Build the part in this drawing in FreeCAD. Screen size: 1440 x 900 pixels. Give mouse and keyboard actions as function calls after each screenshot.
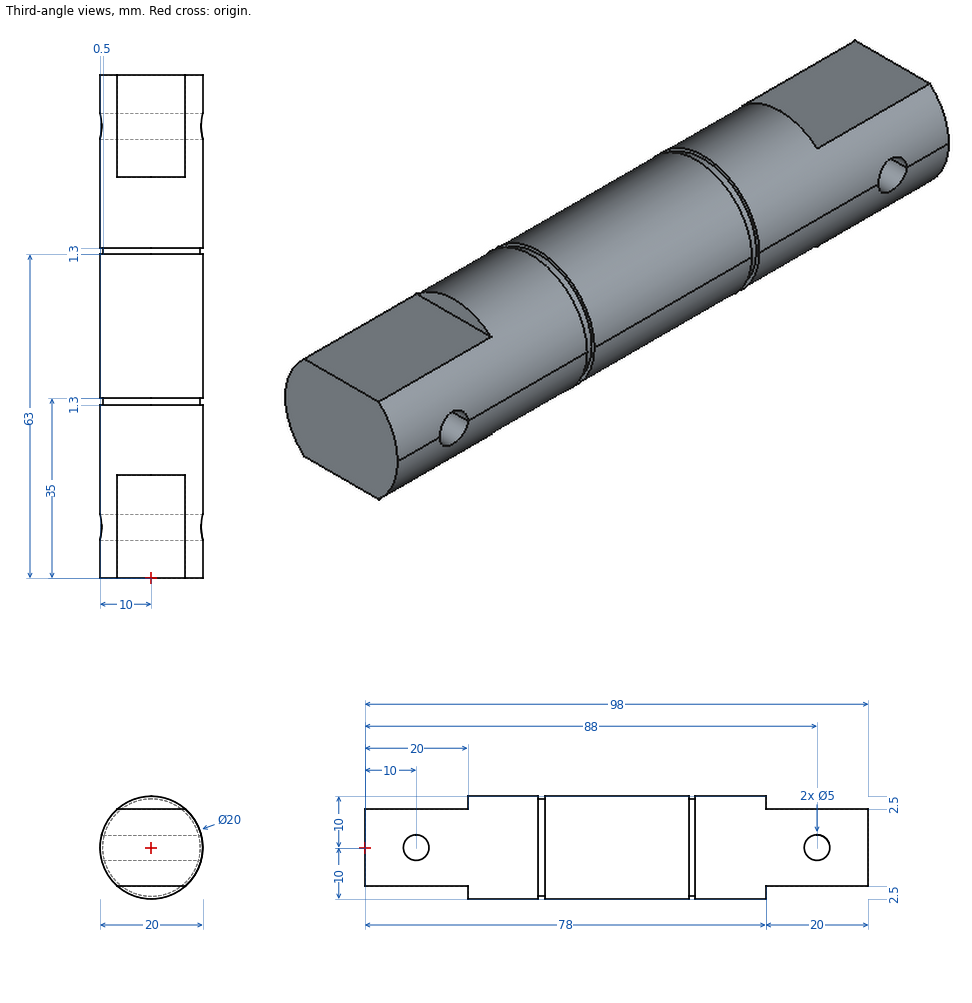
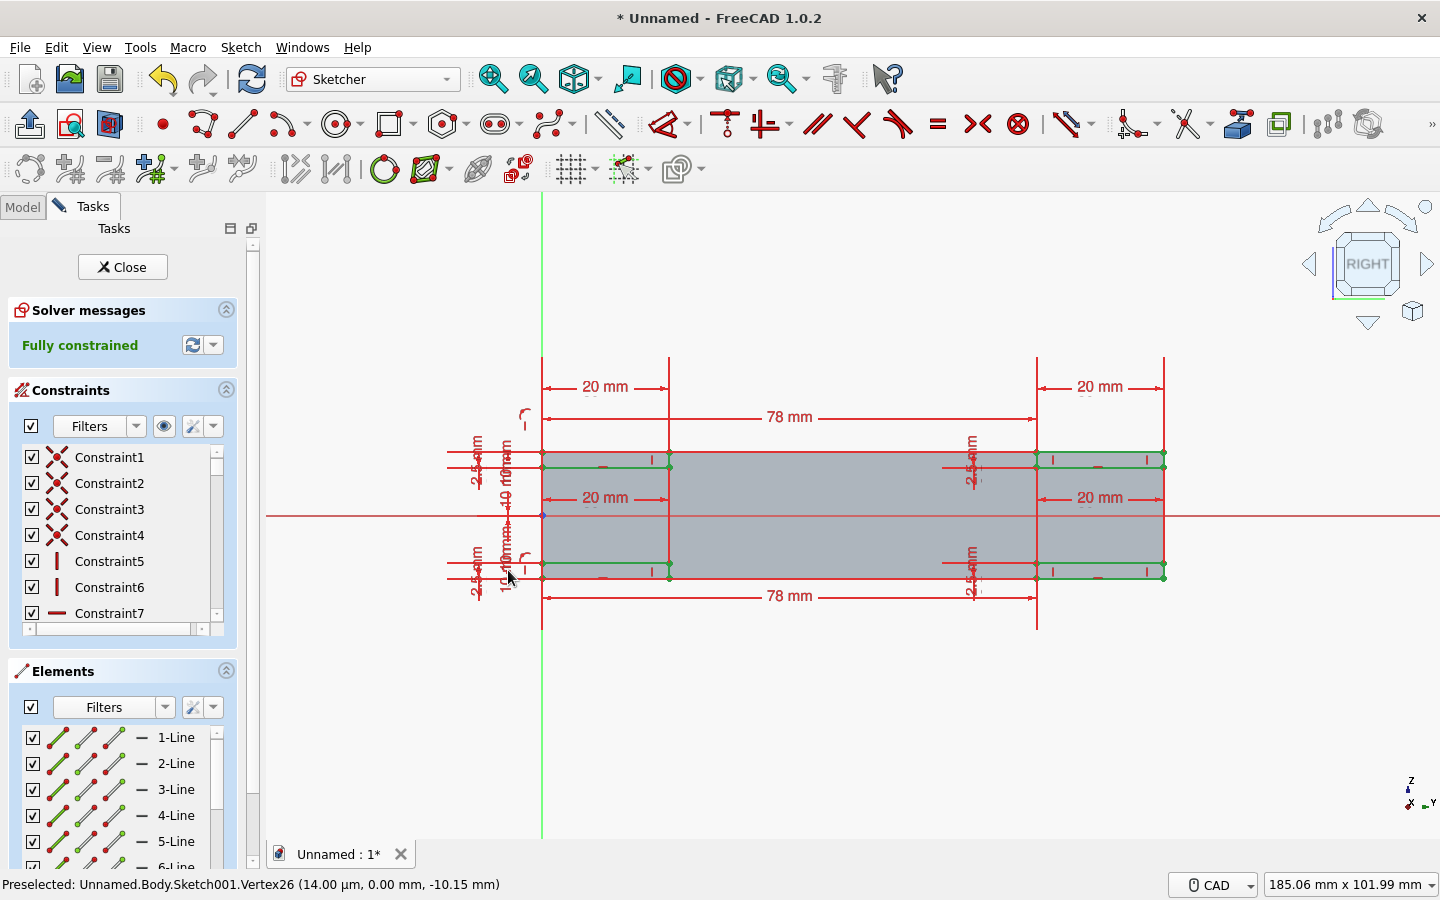
click(123, 267)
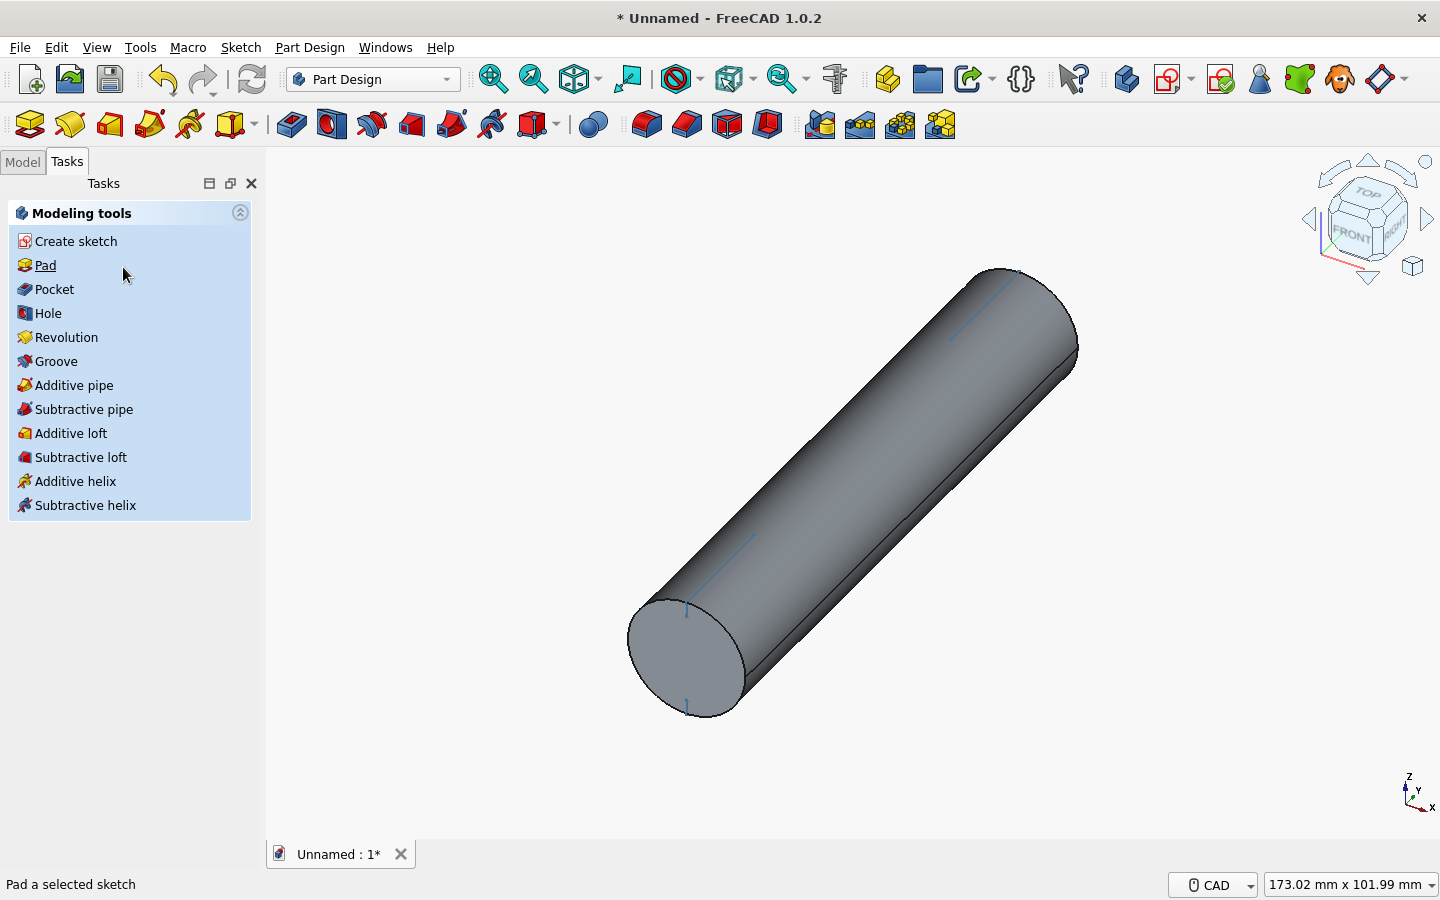
click(292, 124)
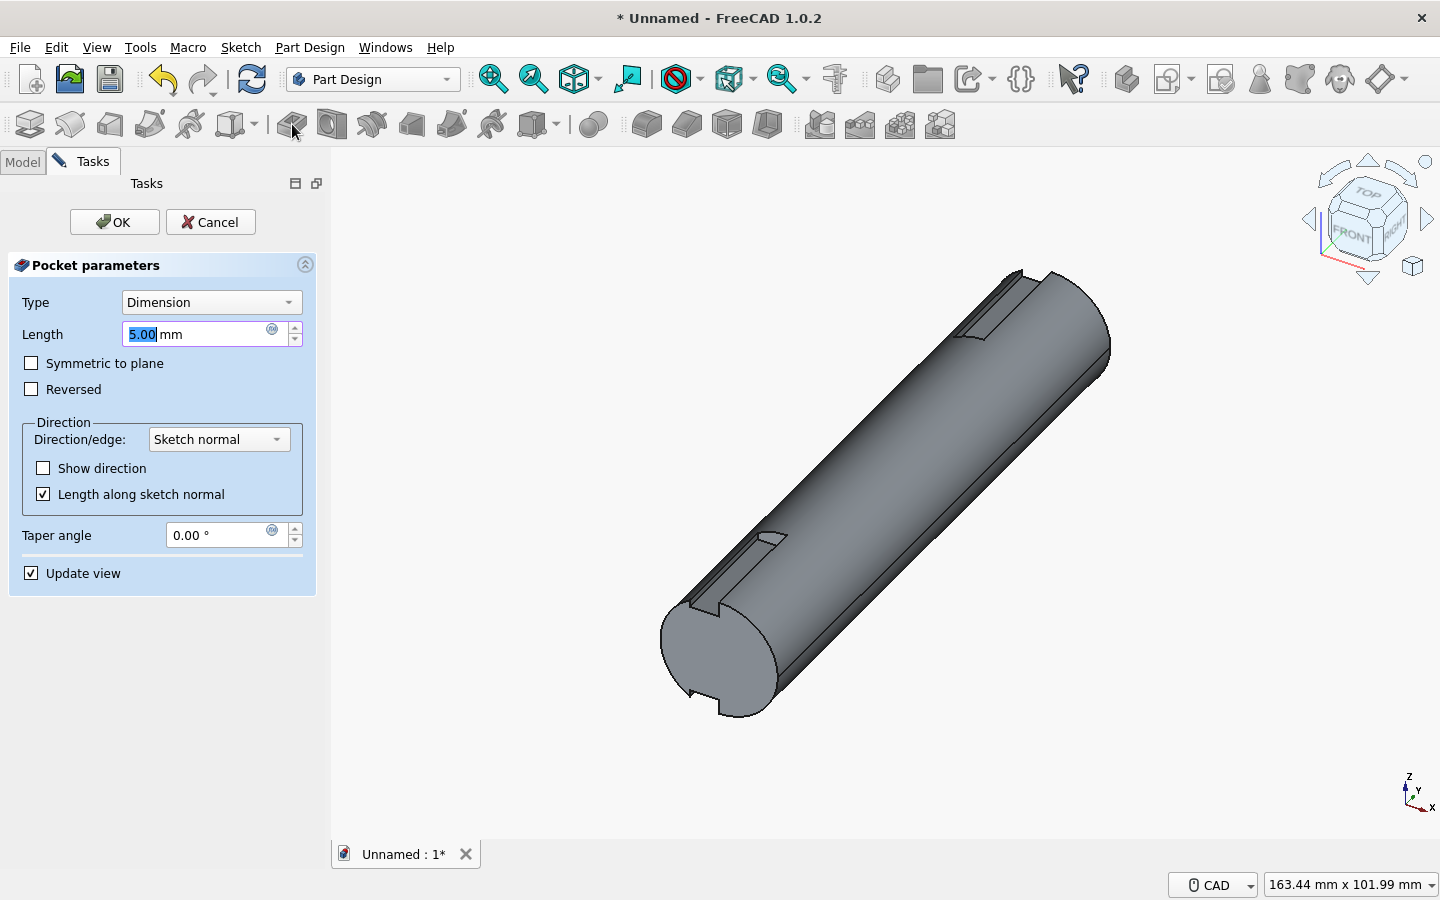
text(20)
key(Tab)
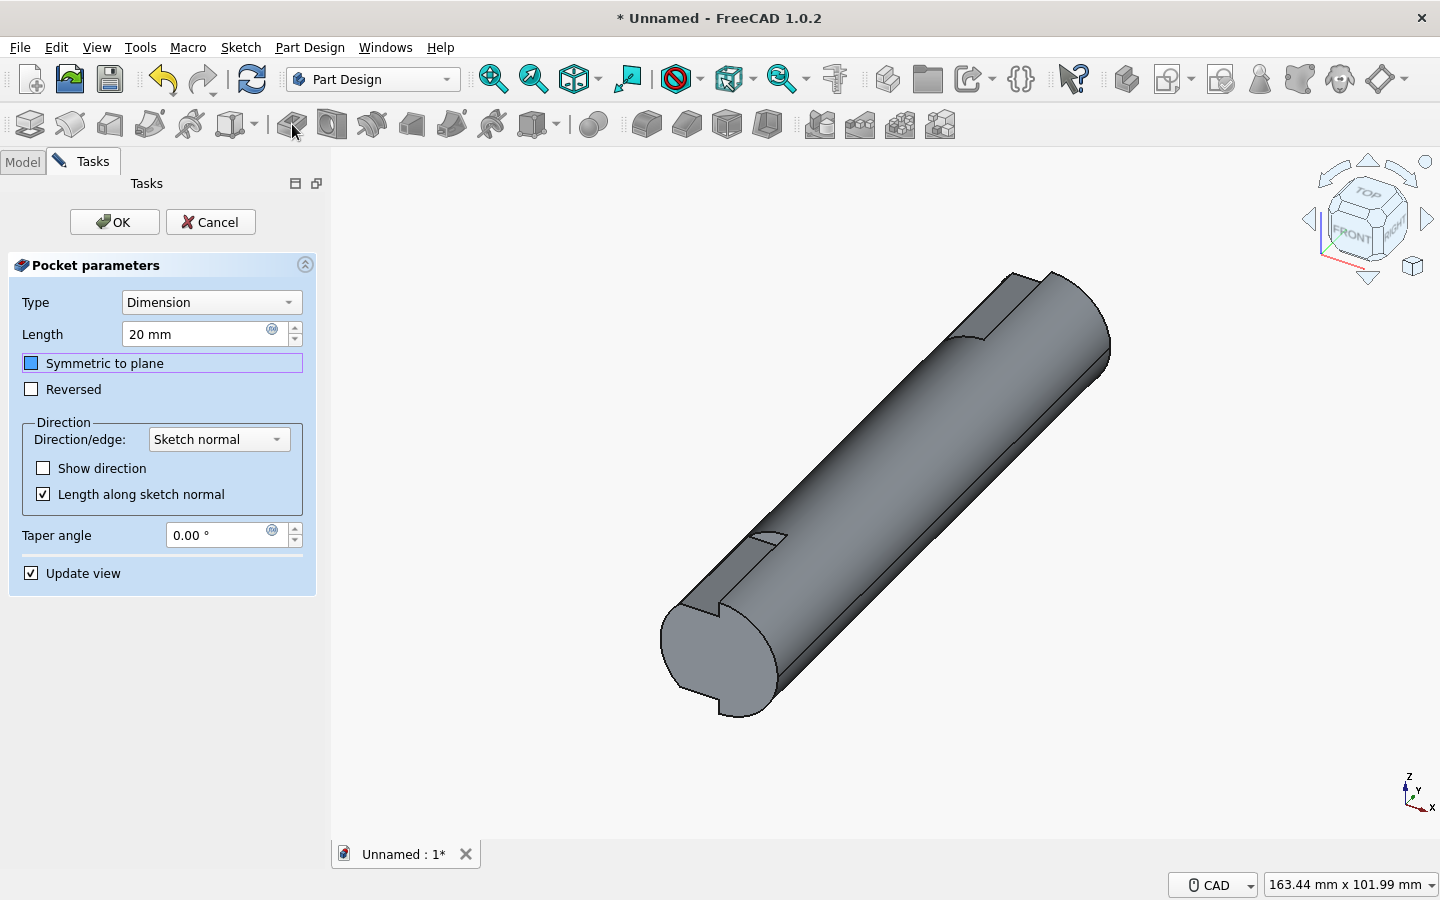
click(30, 363)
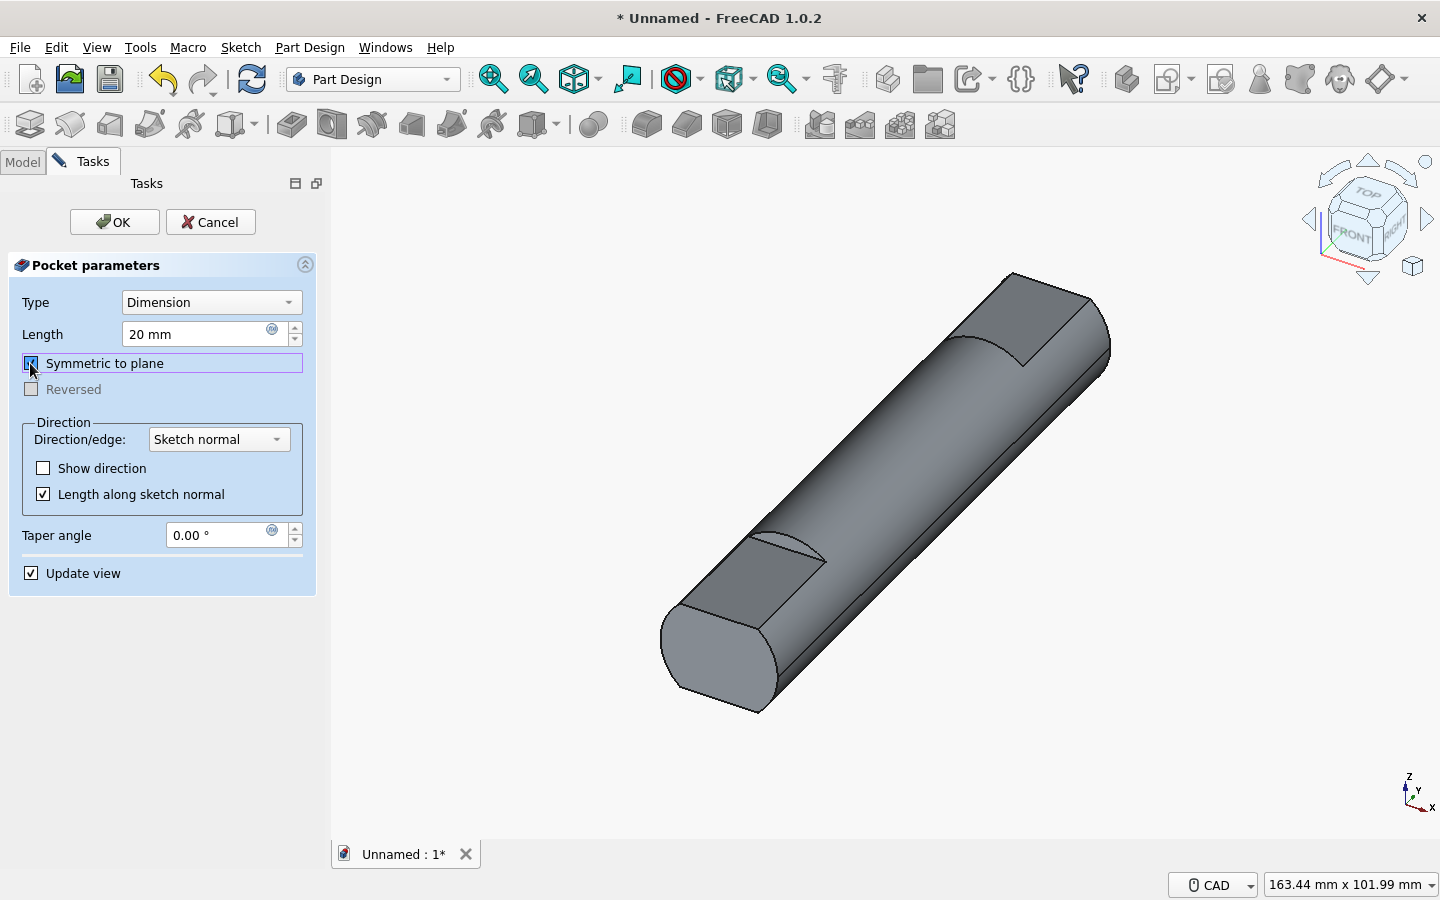
click(115, 222)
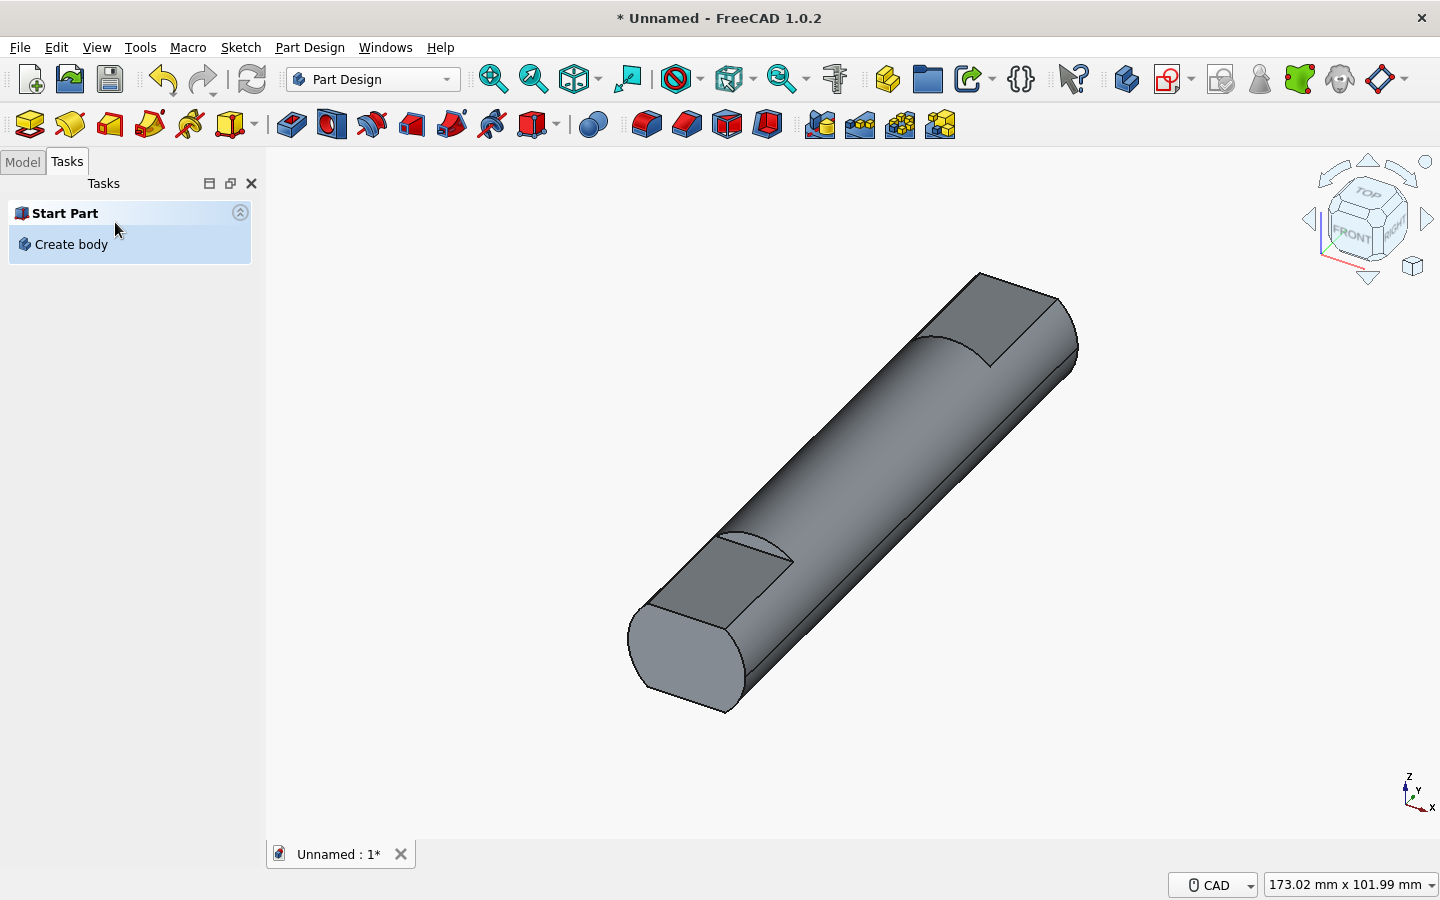
click(23, 161)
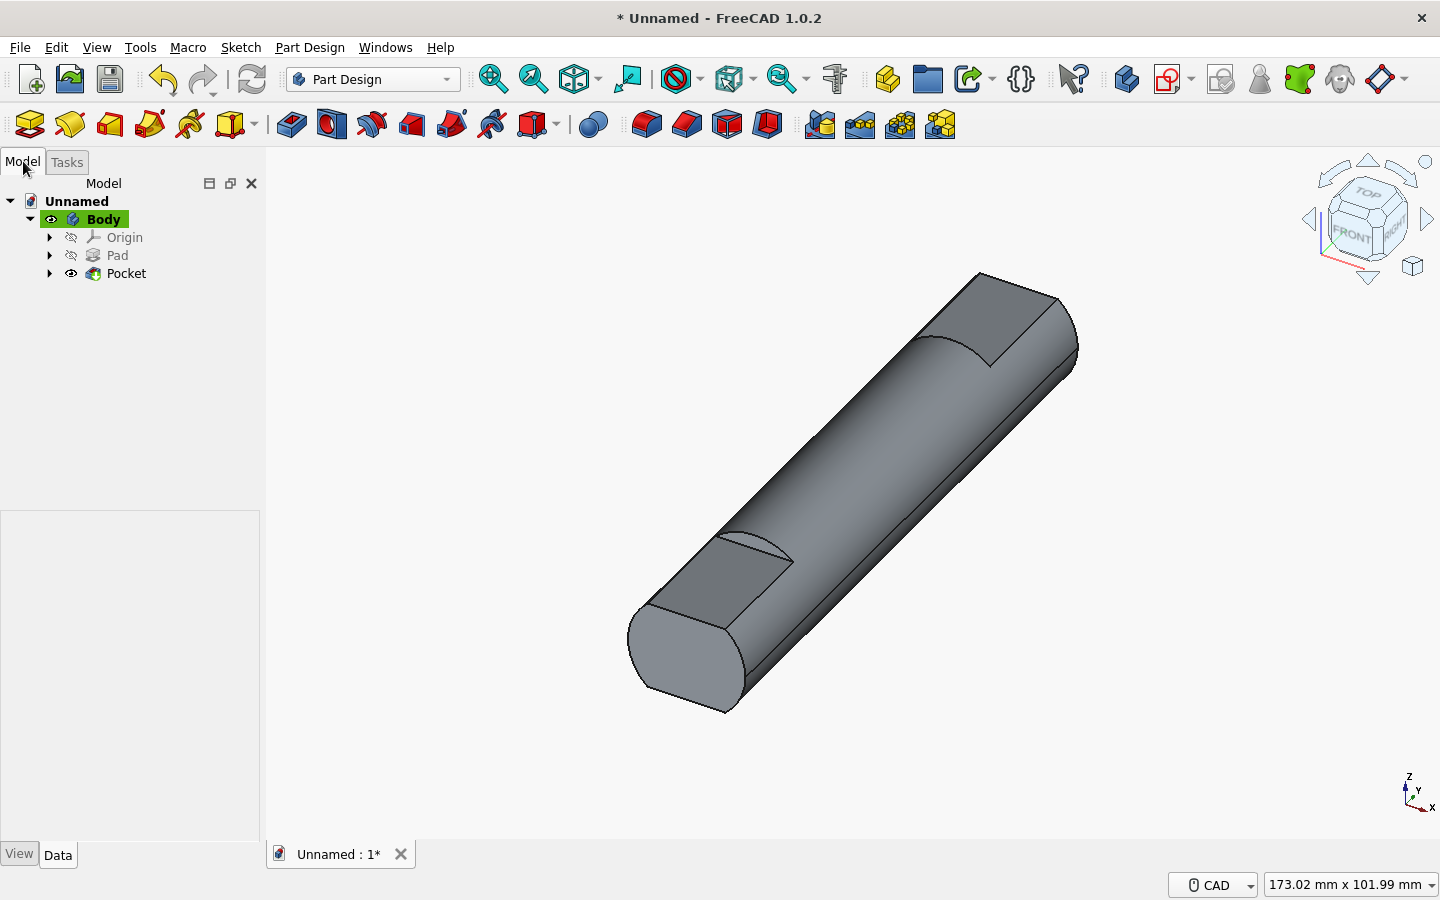
click(50, 237)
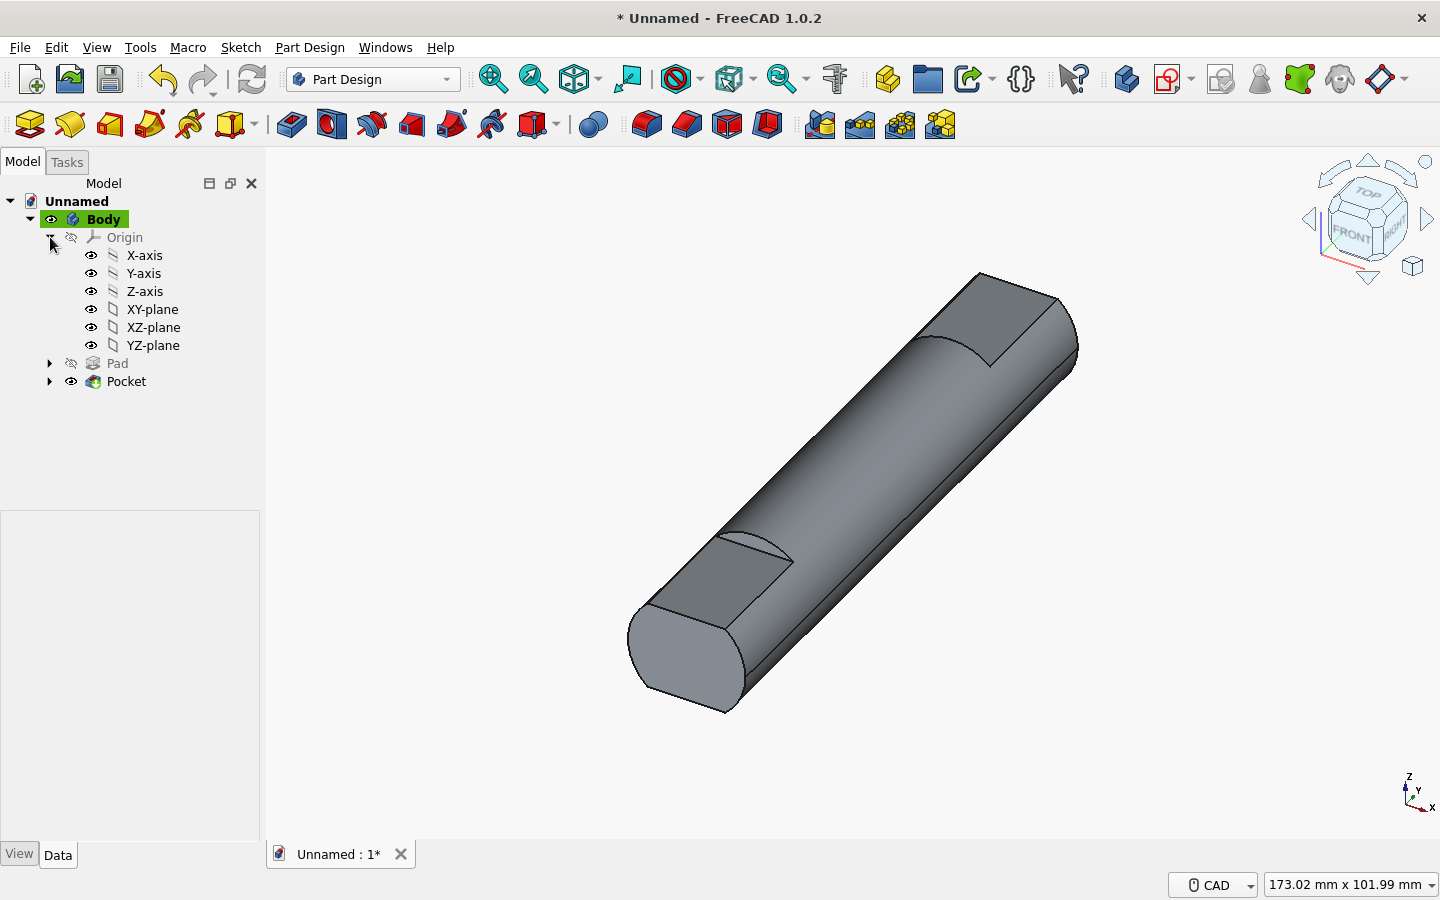
click(136, 345)